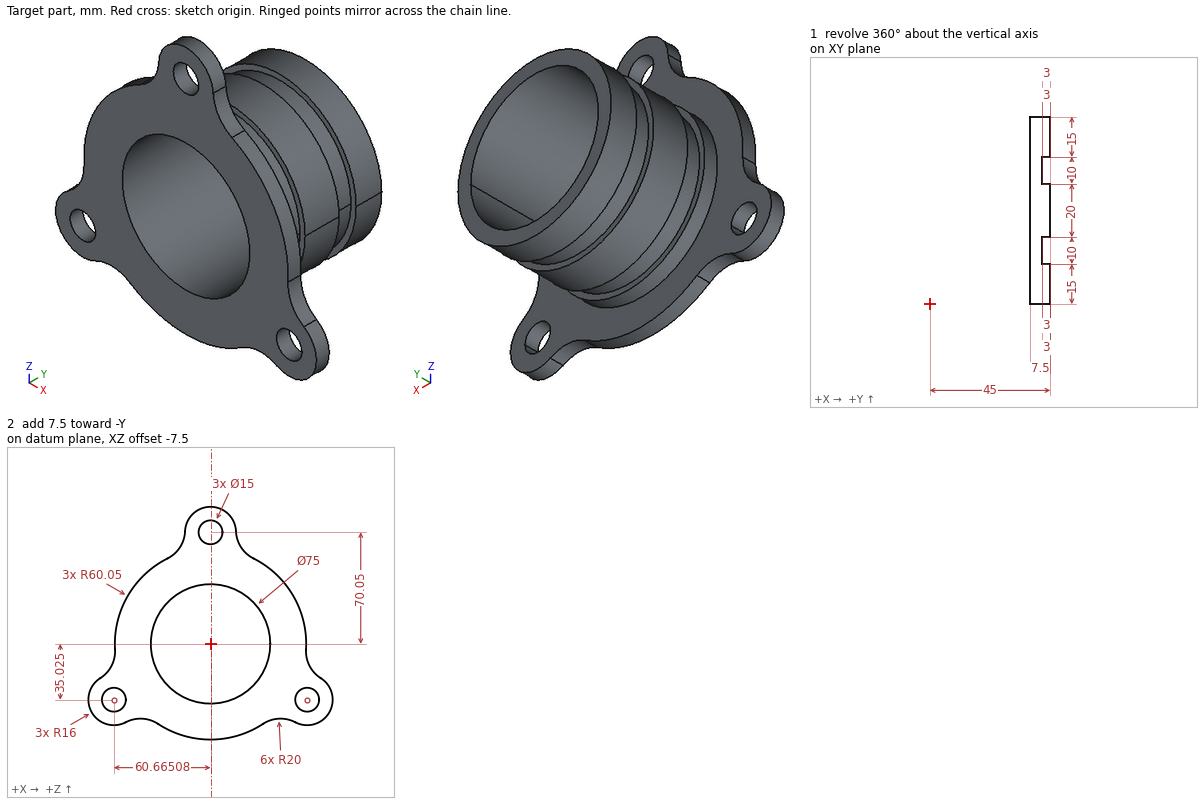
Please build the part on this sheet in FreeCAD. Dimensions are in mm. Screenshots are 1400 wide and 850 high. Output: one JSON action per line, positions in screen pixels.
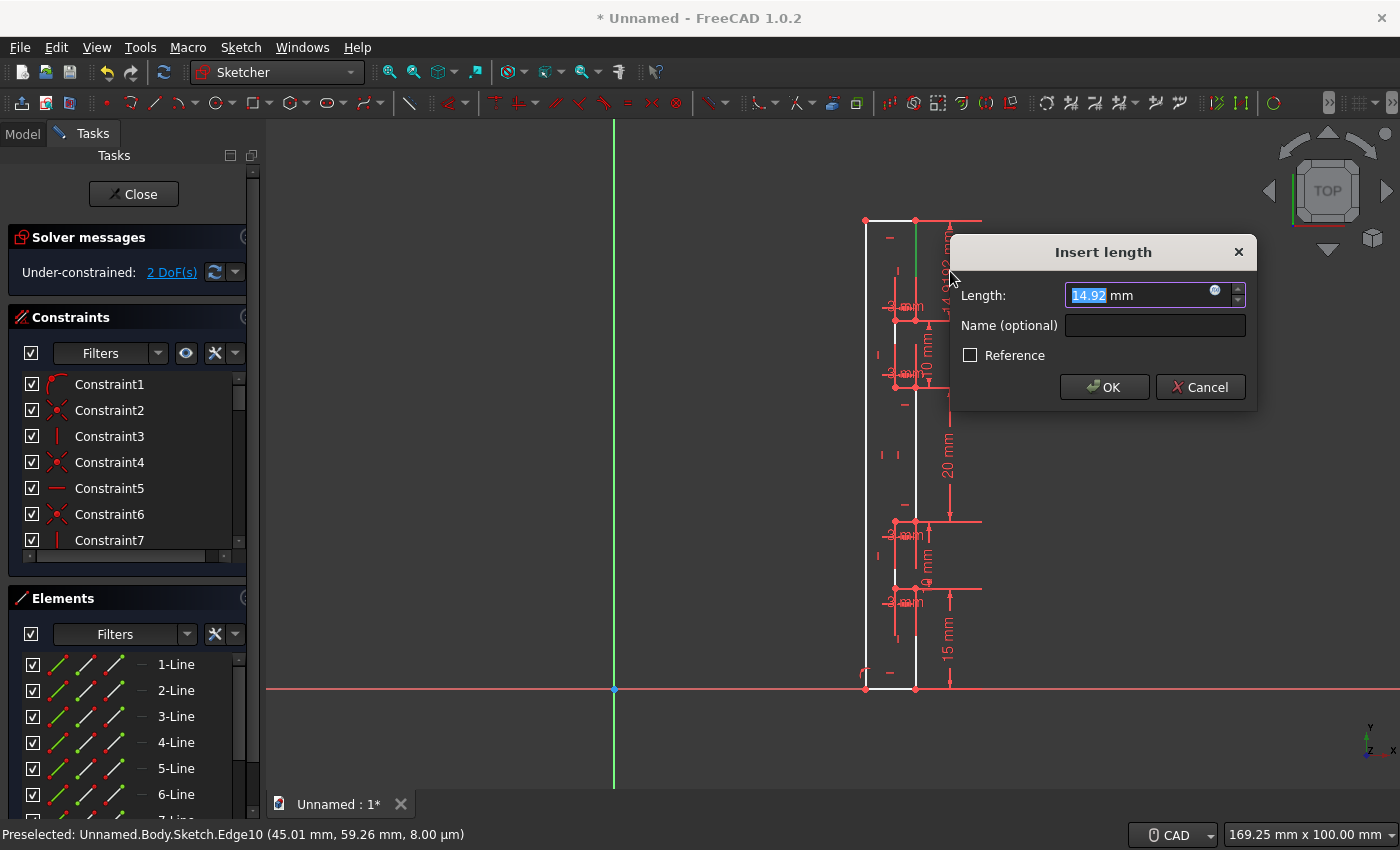
{"action": "type", "text": "15"}
{"action": "key", "text": "Return"}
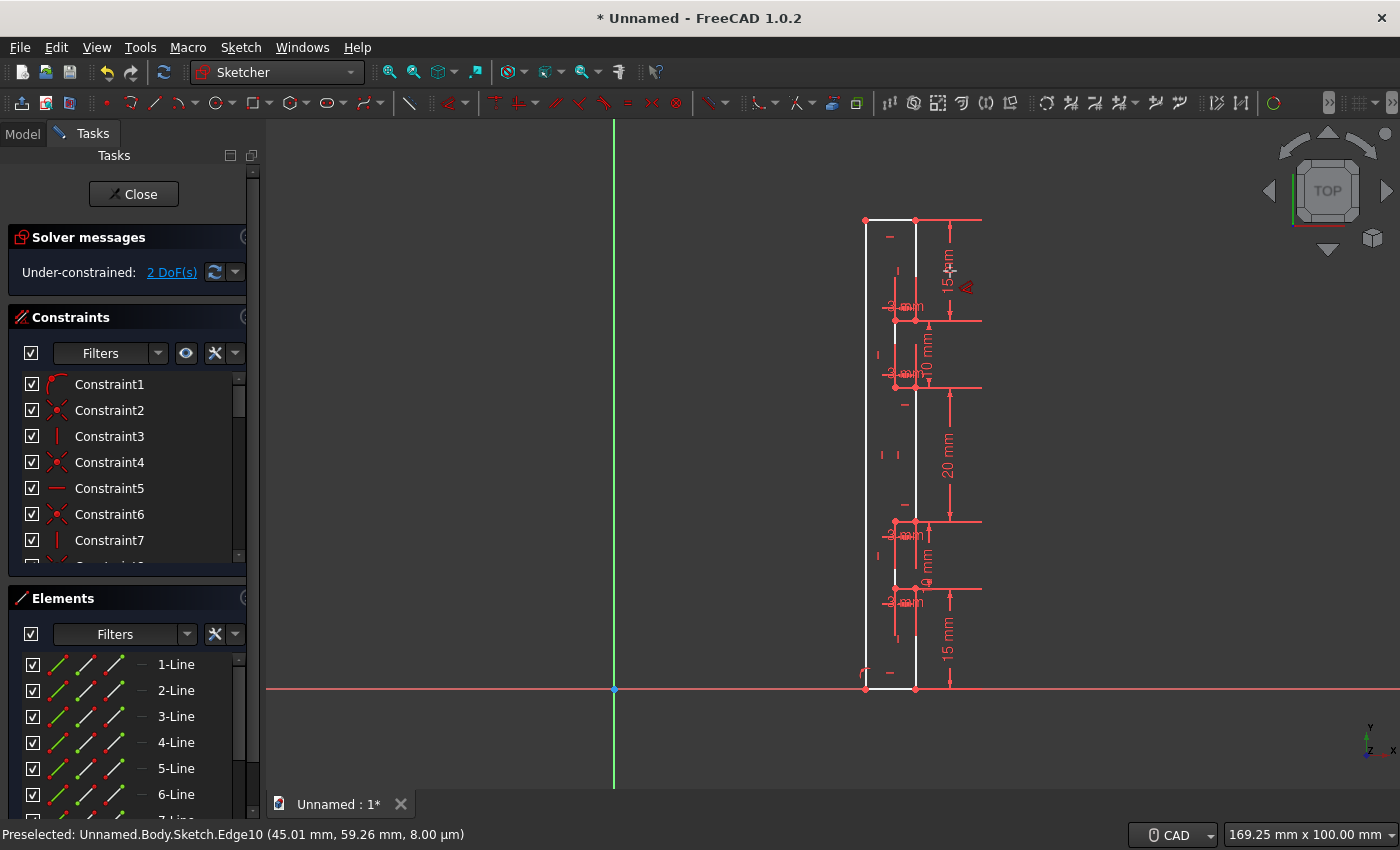
{"action": "left_click", "coordinate": [881, 689]}
{"action": "left_click", "coordinate": [891, 723]}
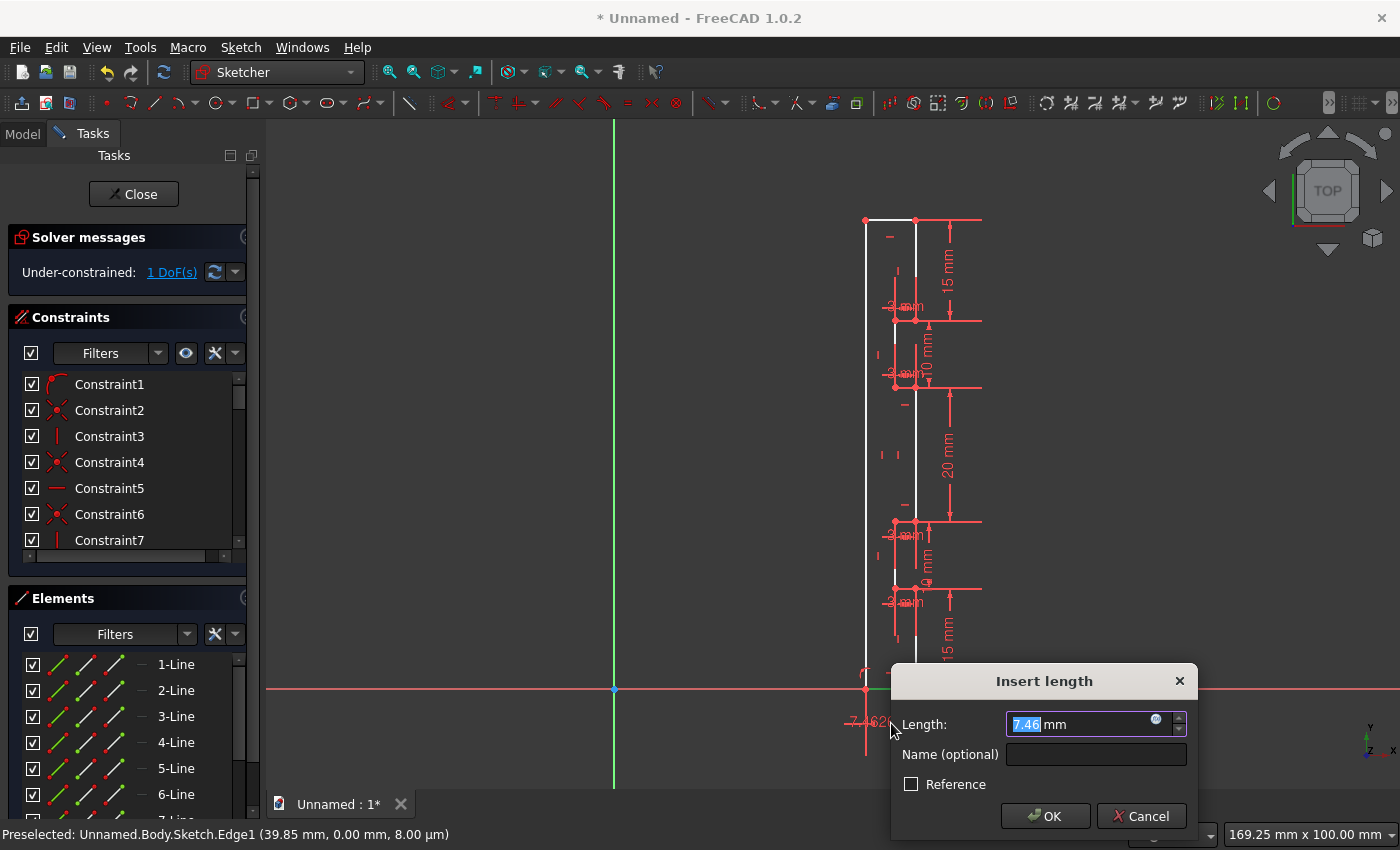
{"action": "type", "text": "7.5"}
{"action": "key", "text": "Return"}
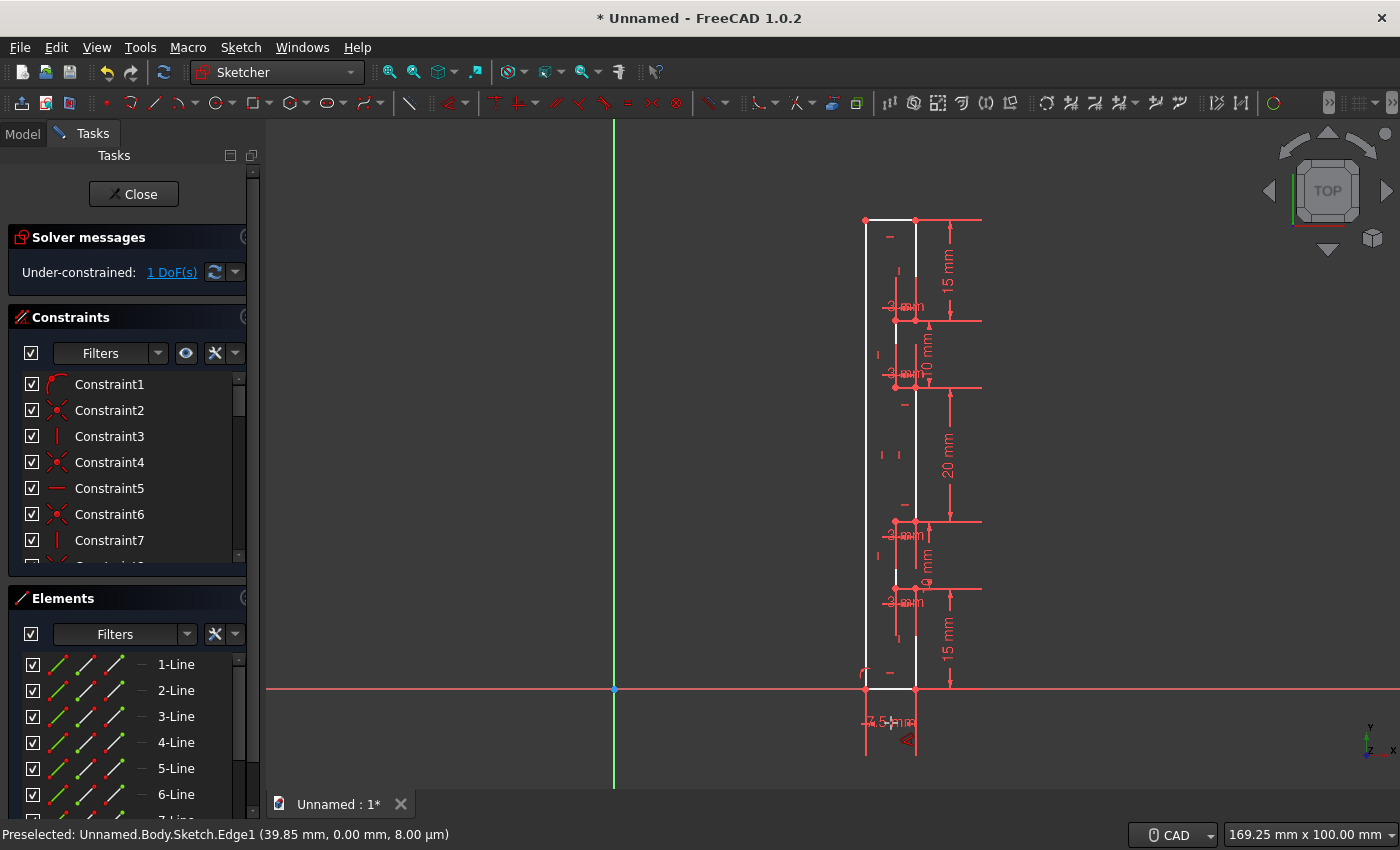
{"action": "left_click", "coordinate": [916, 689]}
{"action": "left_click", "coordinate": [765, 723]}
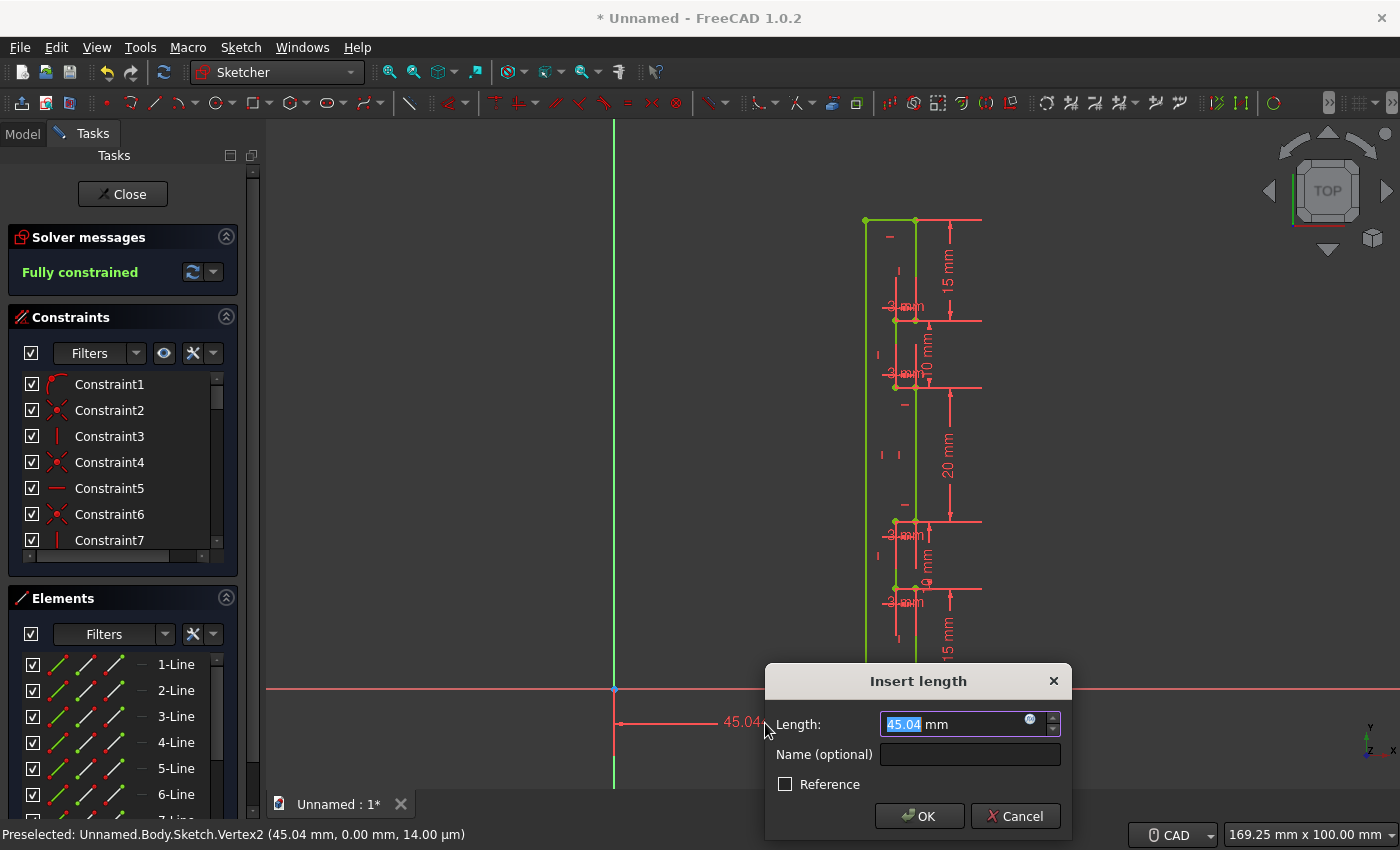
{"action": "type", "text": "45"}
{"action": "key", "text": "Return"}
{"action": "key", "text": "Escape"}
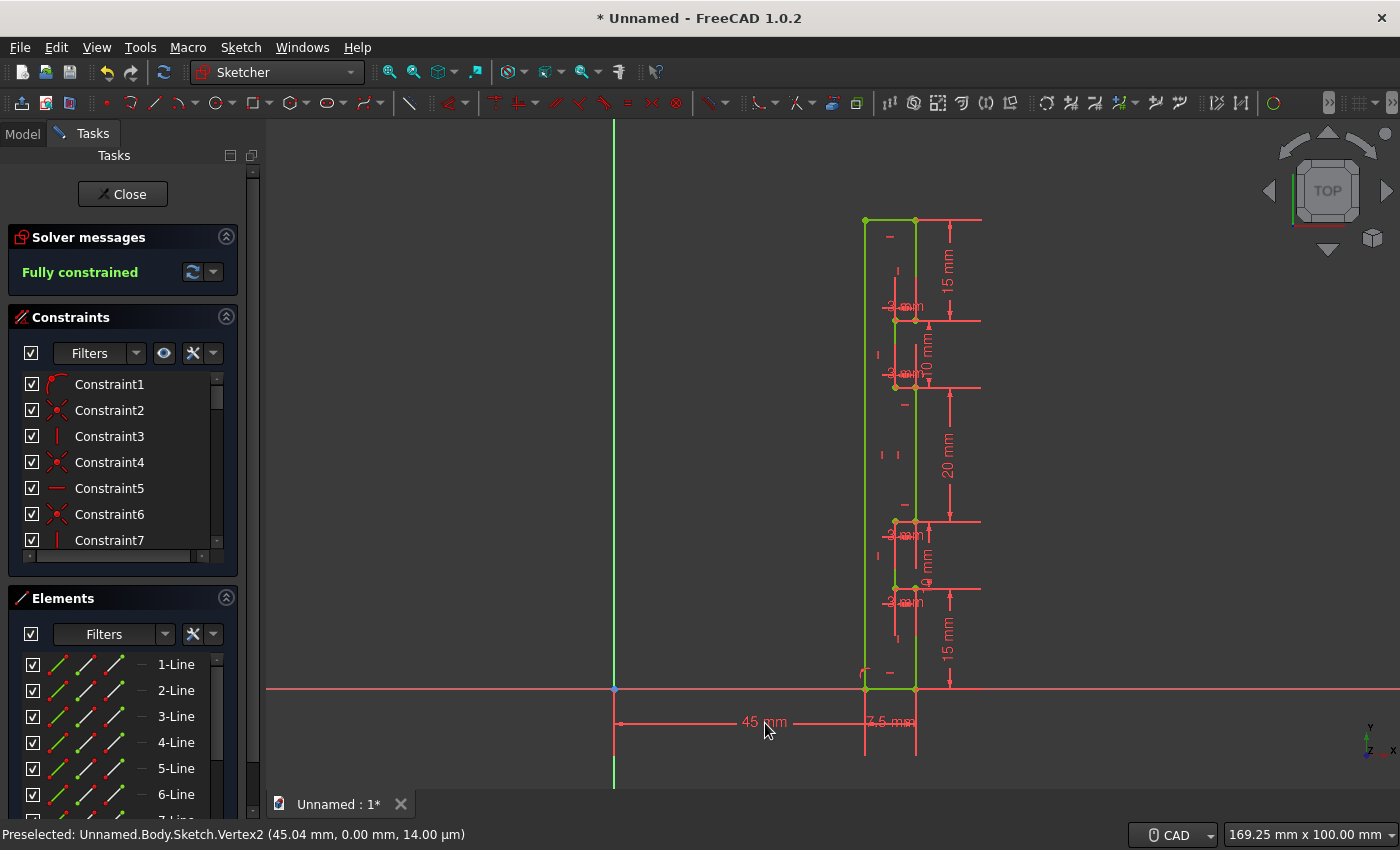
{"action": "left_click", "coordinate": [123, 194]}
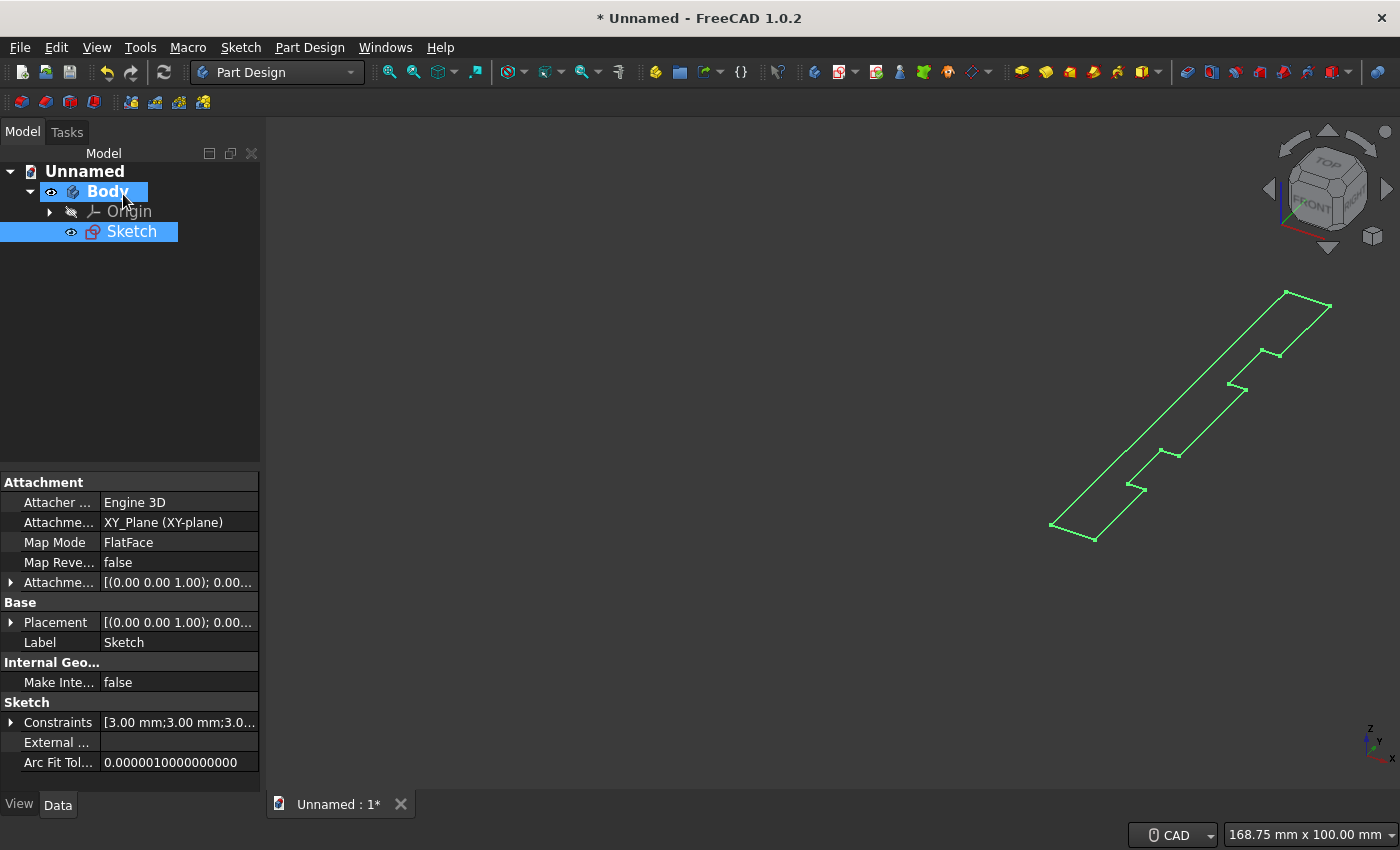
{"action": "left_click", "coordinate": [1046, 72]}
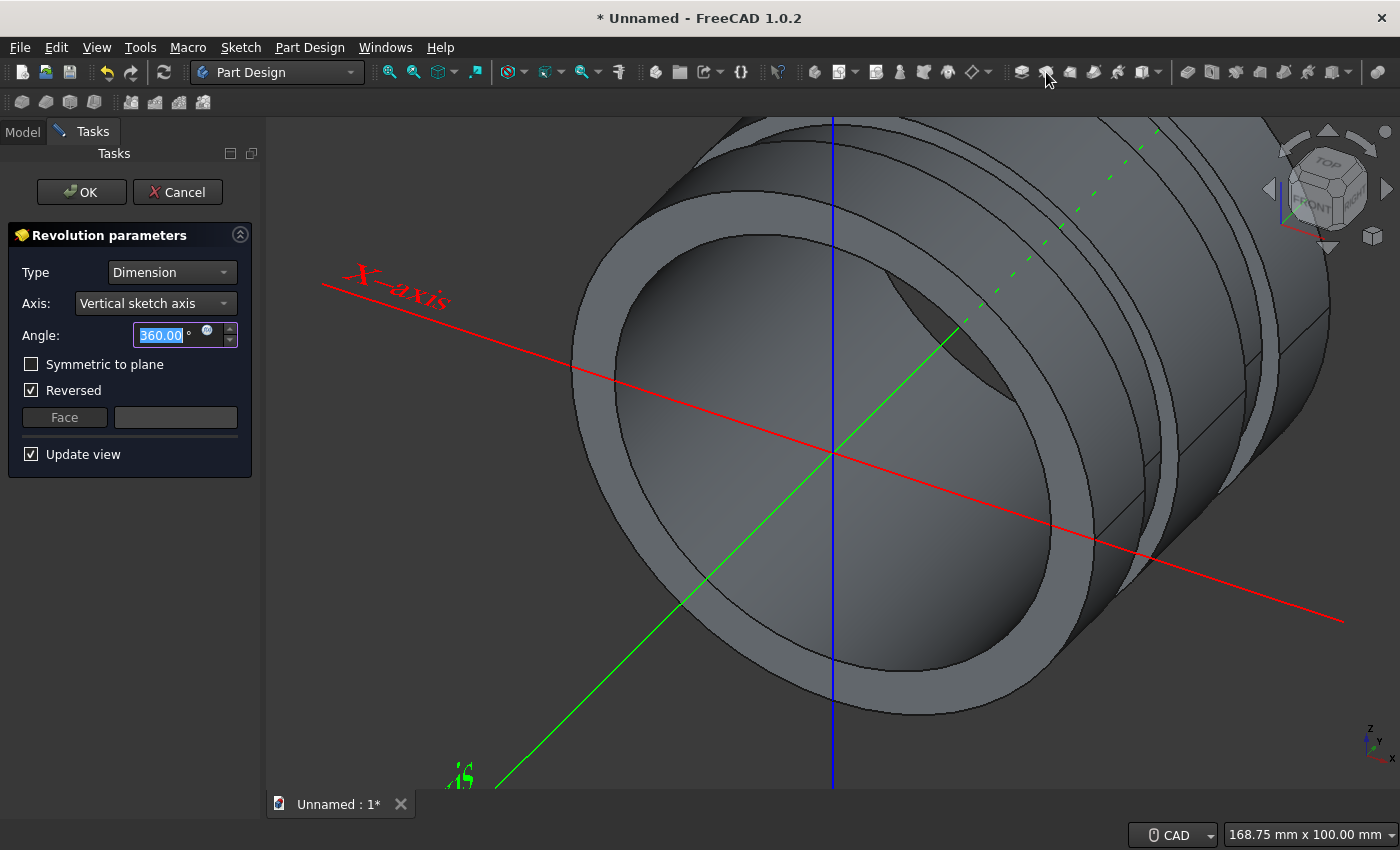
{"action": "left_click", "coordinate": [82, 192]}